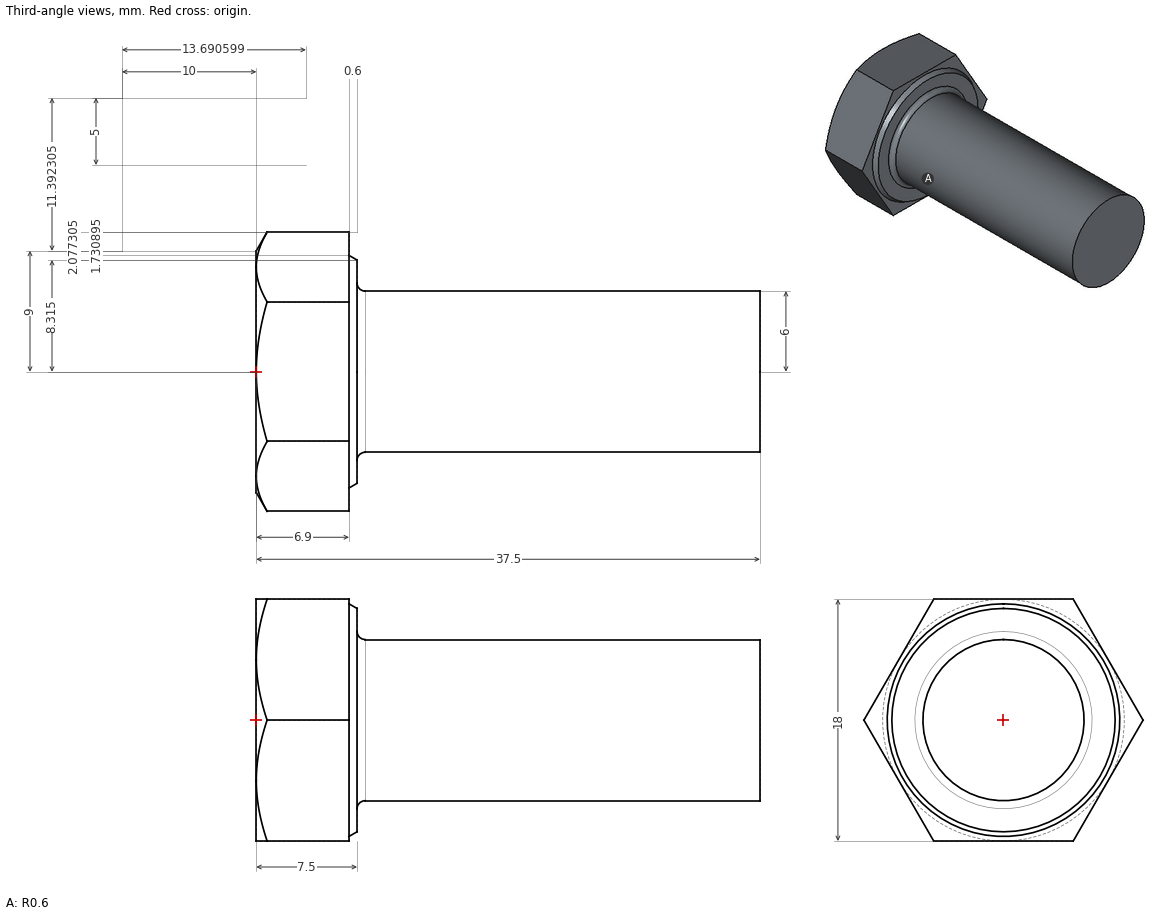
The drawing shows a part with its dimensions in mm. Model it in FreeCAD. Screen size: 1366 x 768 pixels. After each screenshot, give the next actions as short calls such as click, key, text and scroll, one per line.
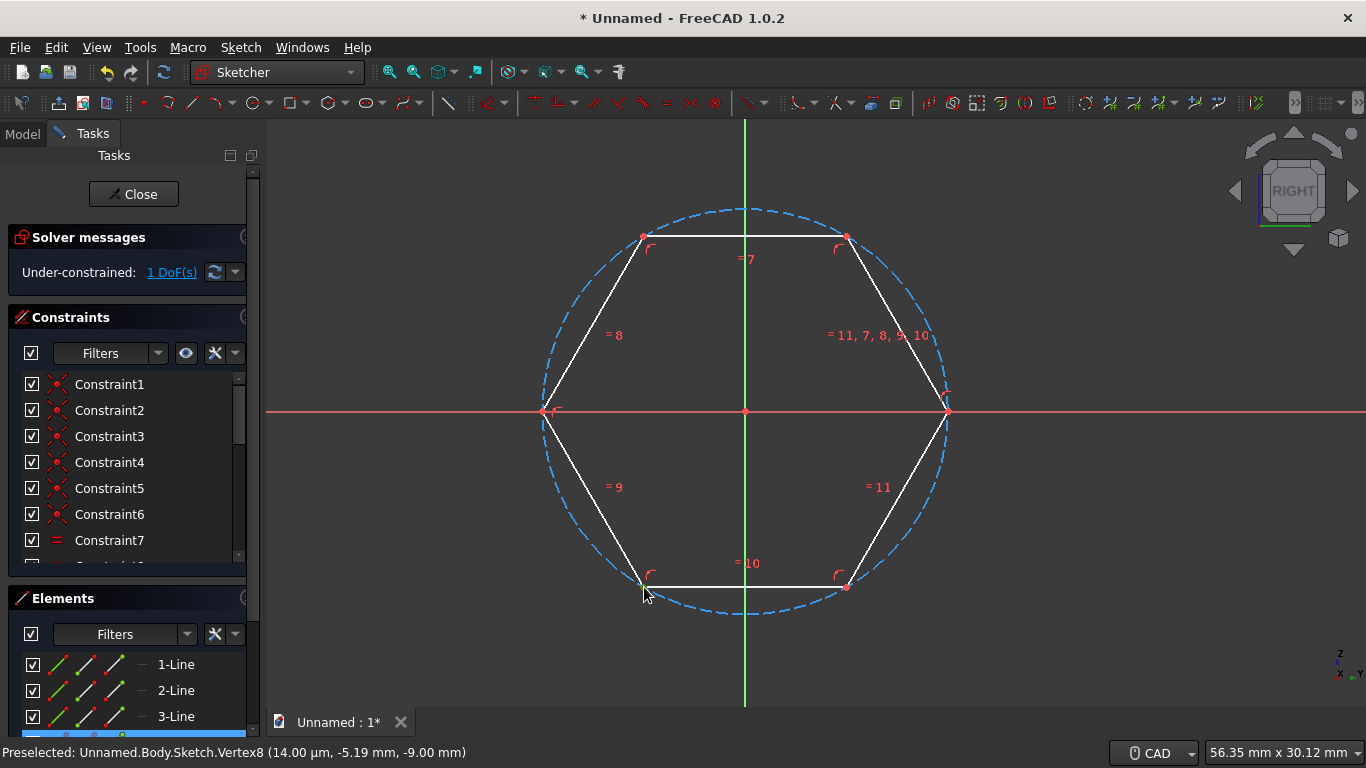
click(847, 236)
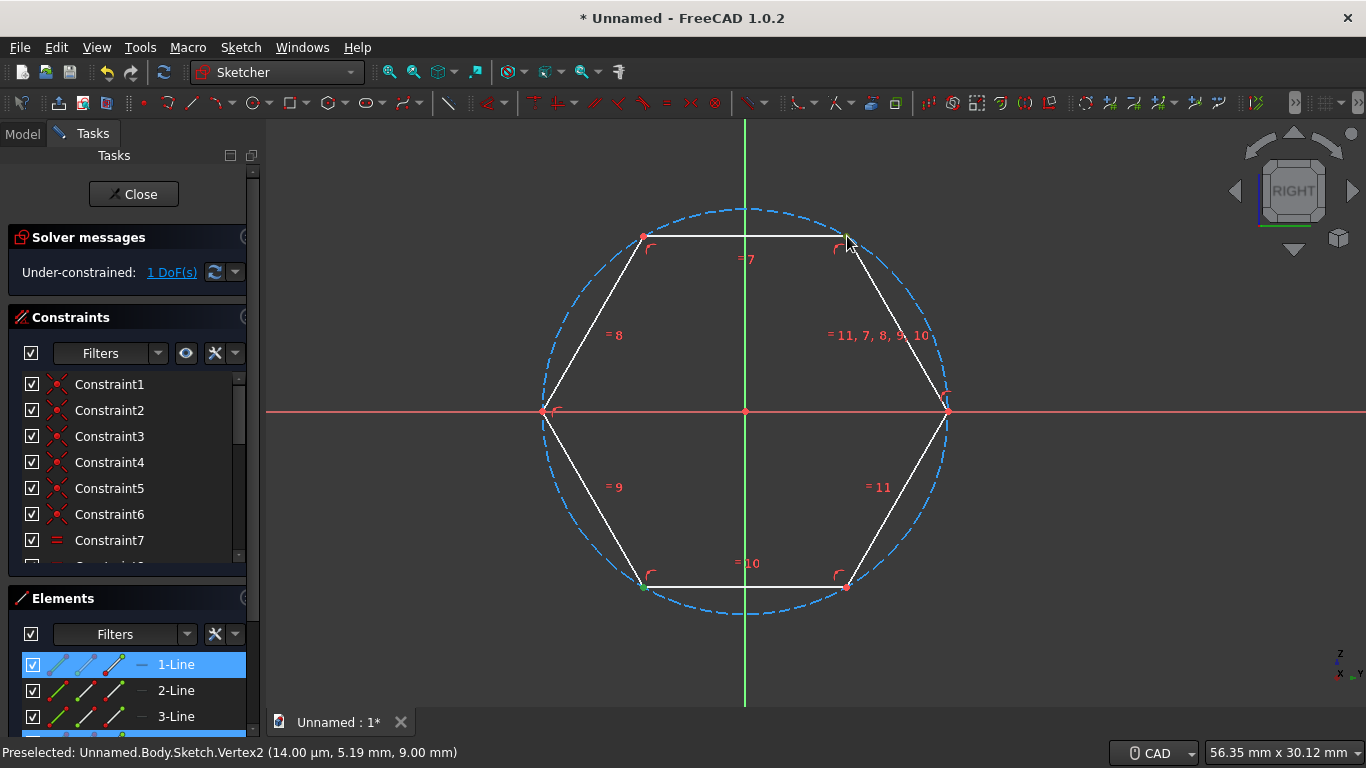
key(i)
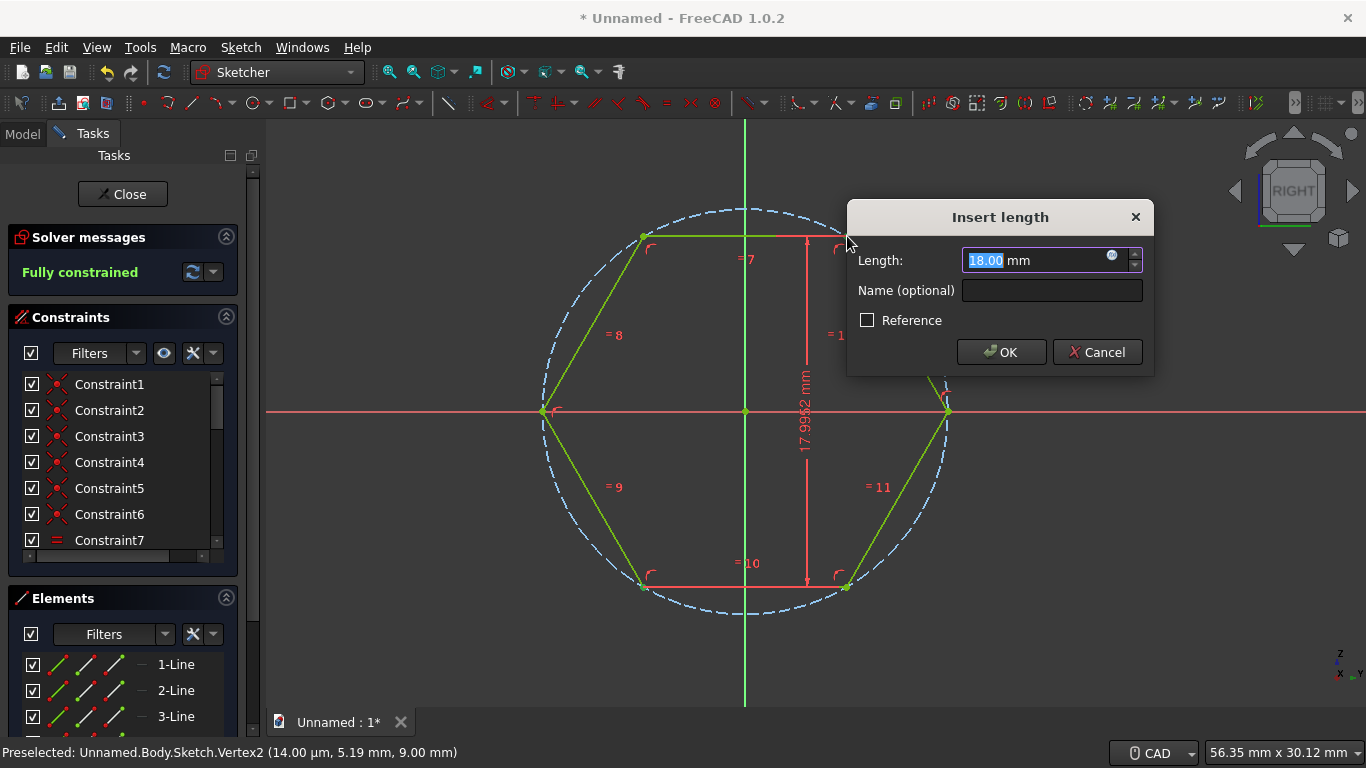
text(18)
key(Return)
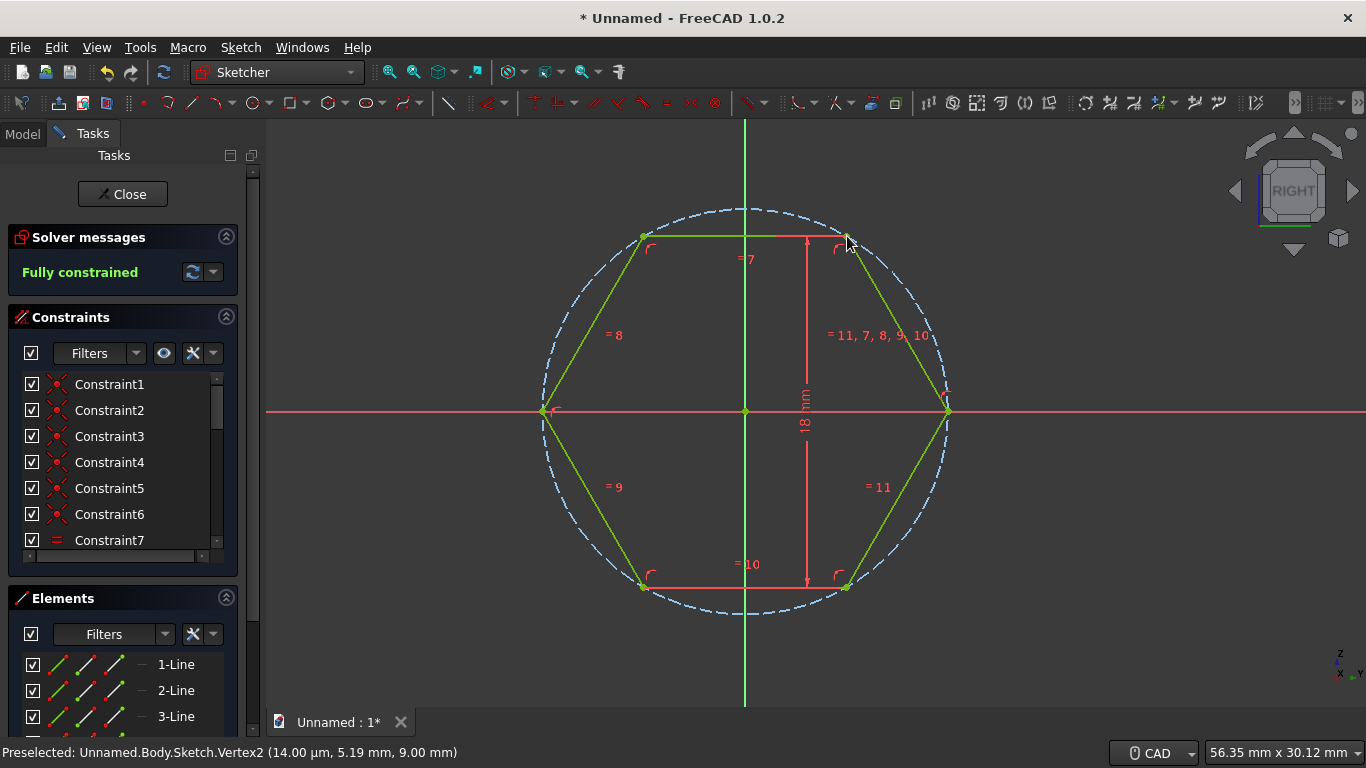
click(123, 194)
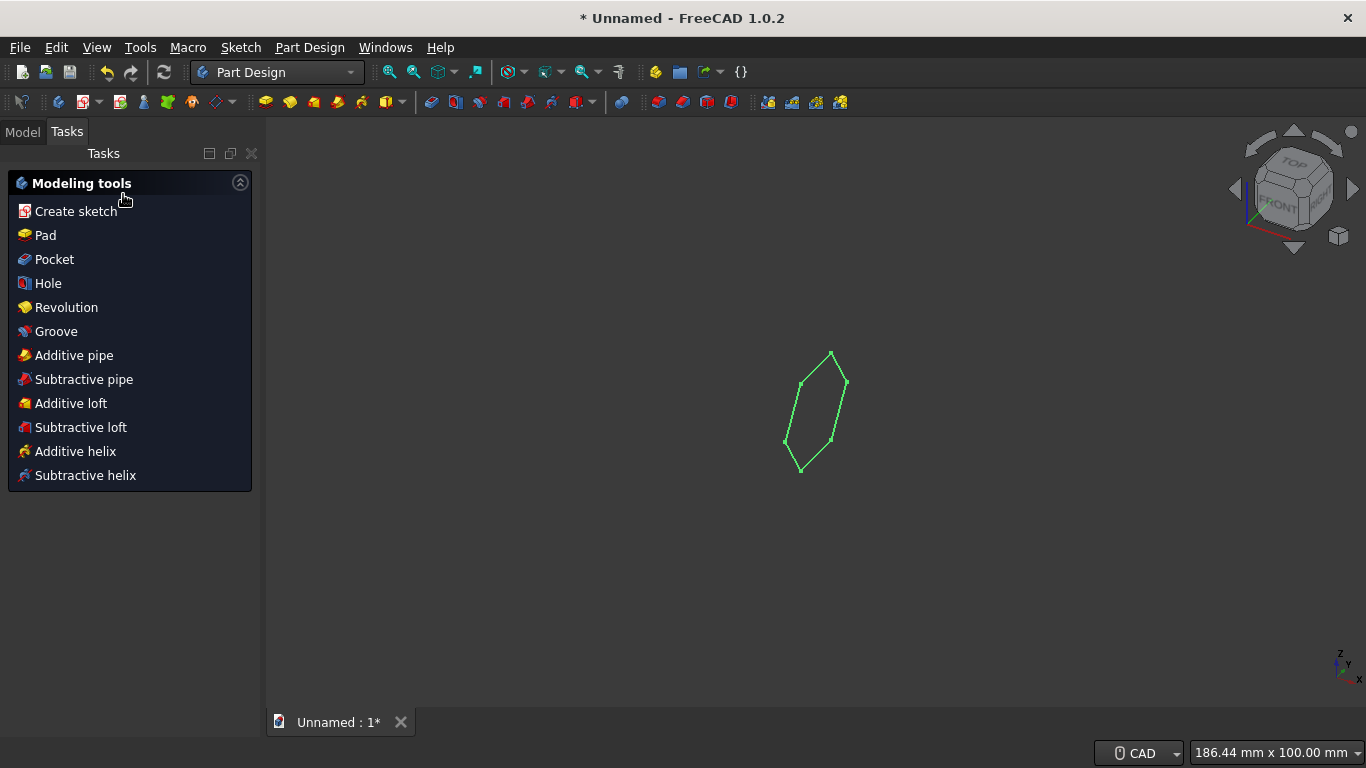
click(266, 102)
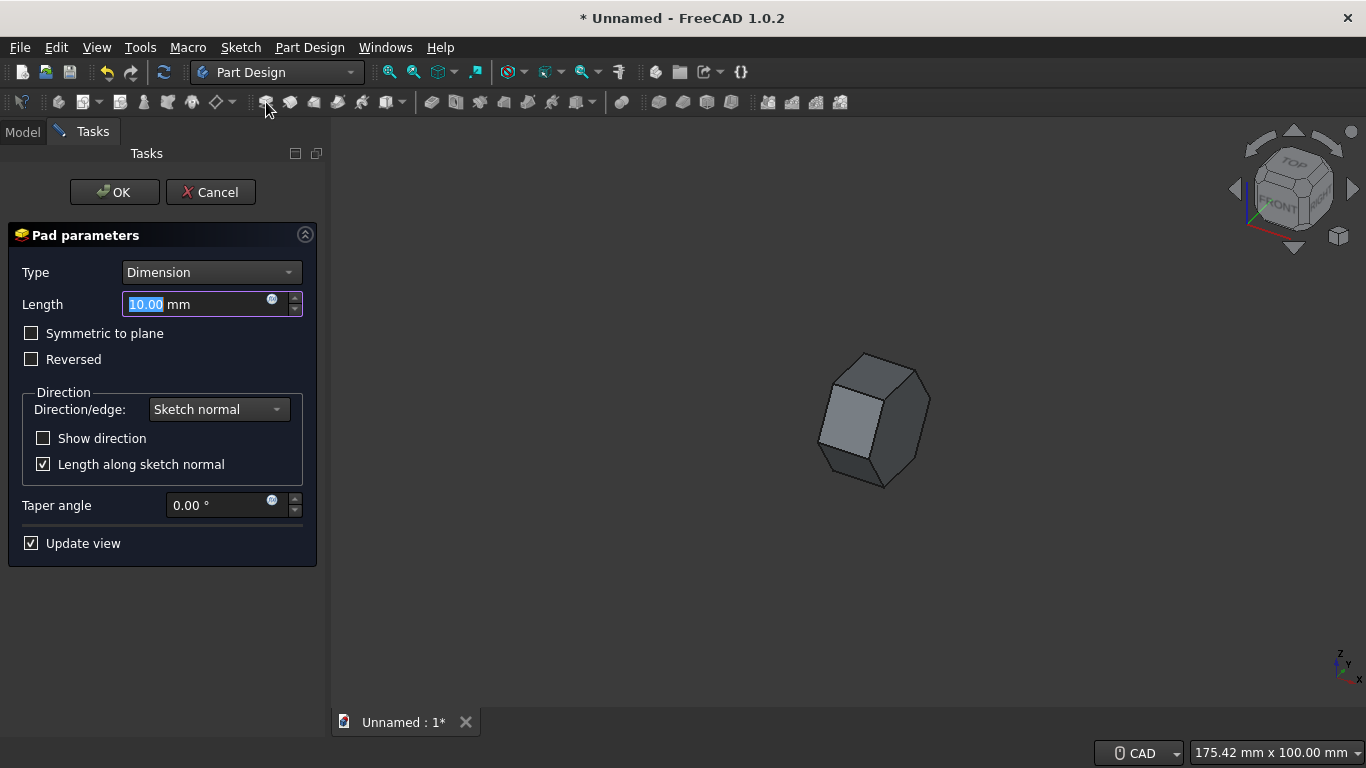
text(7.5)
key(Tab)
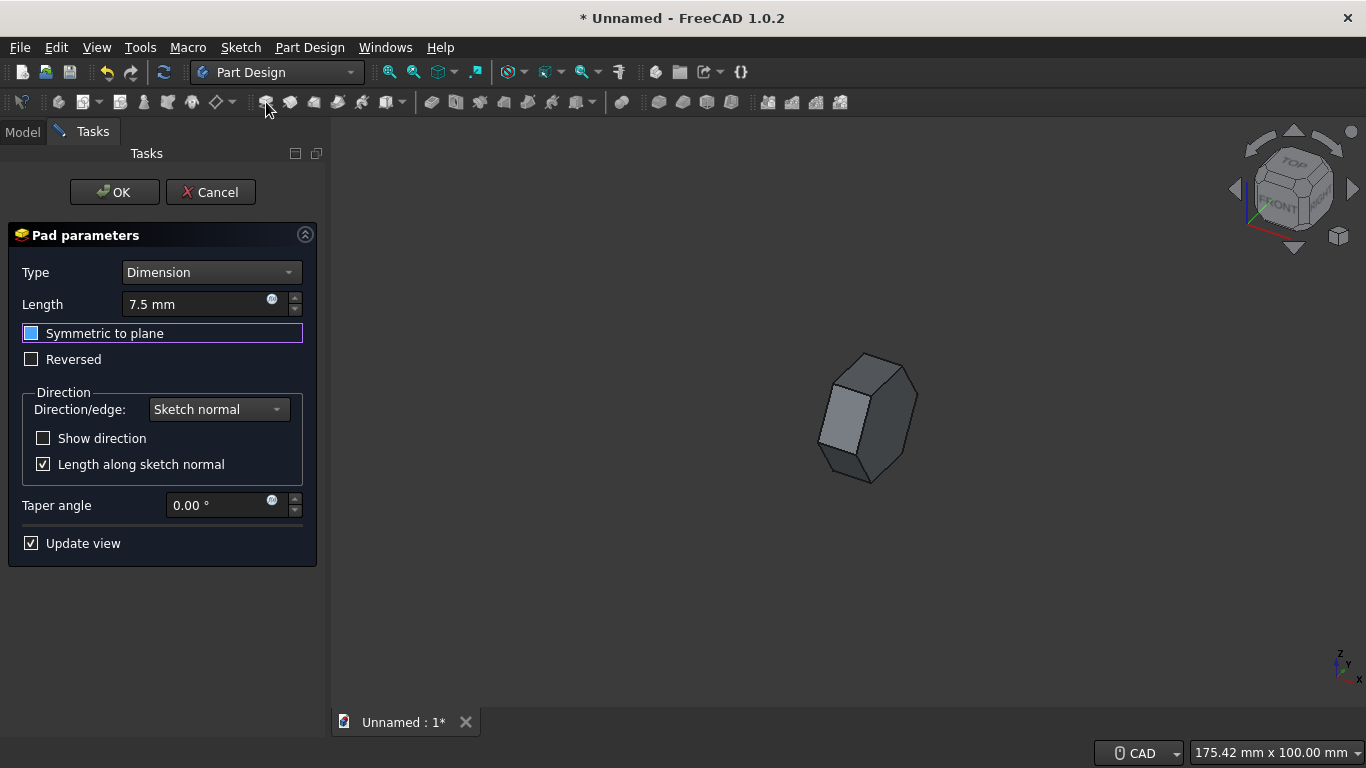
click(115, 192)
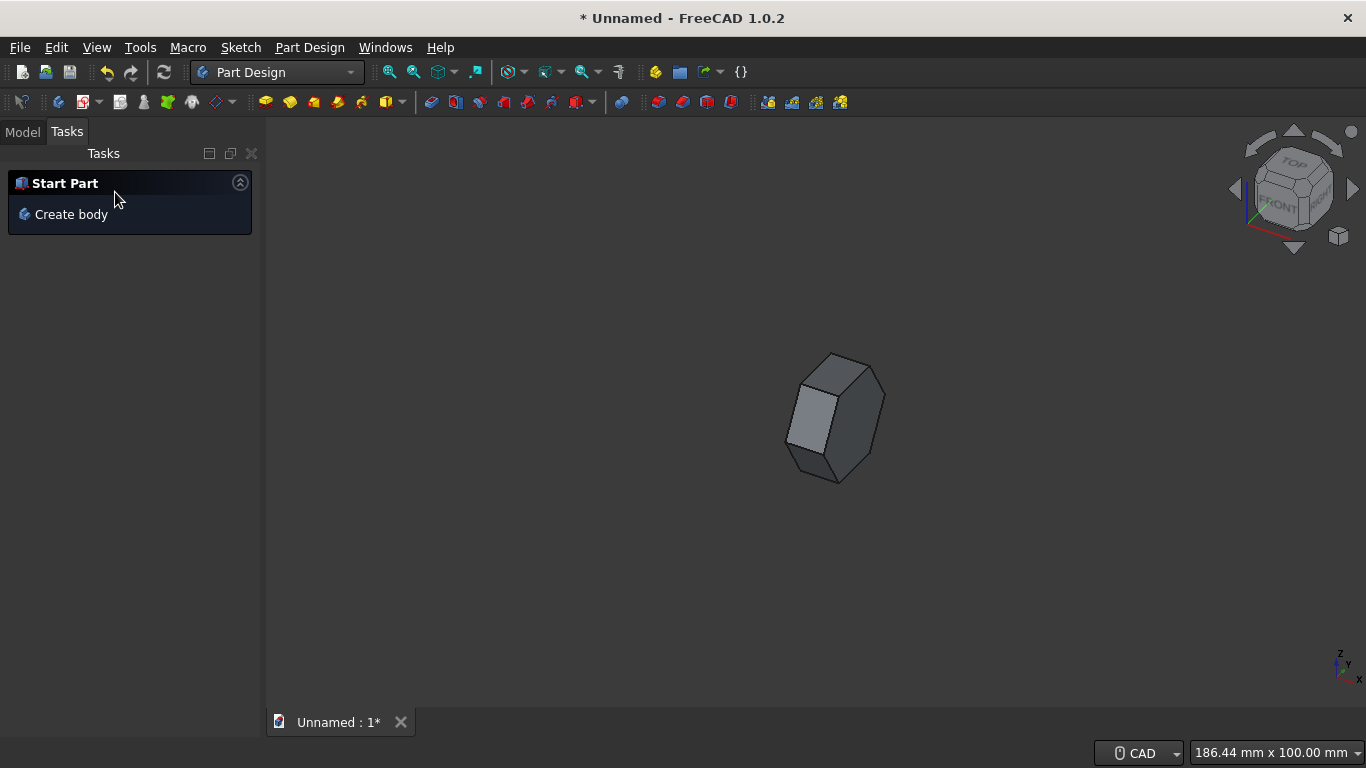
key(v)
key(f)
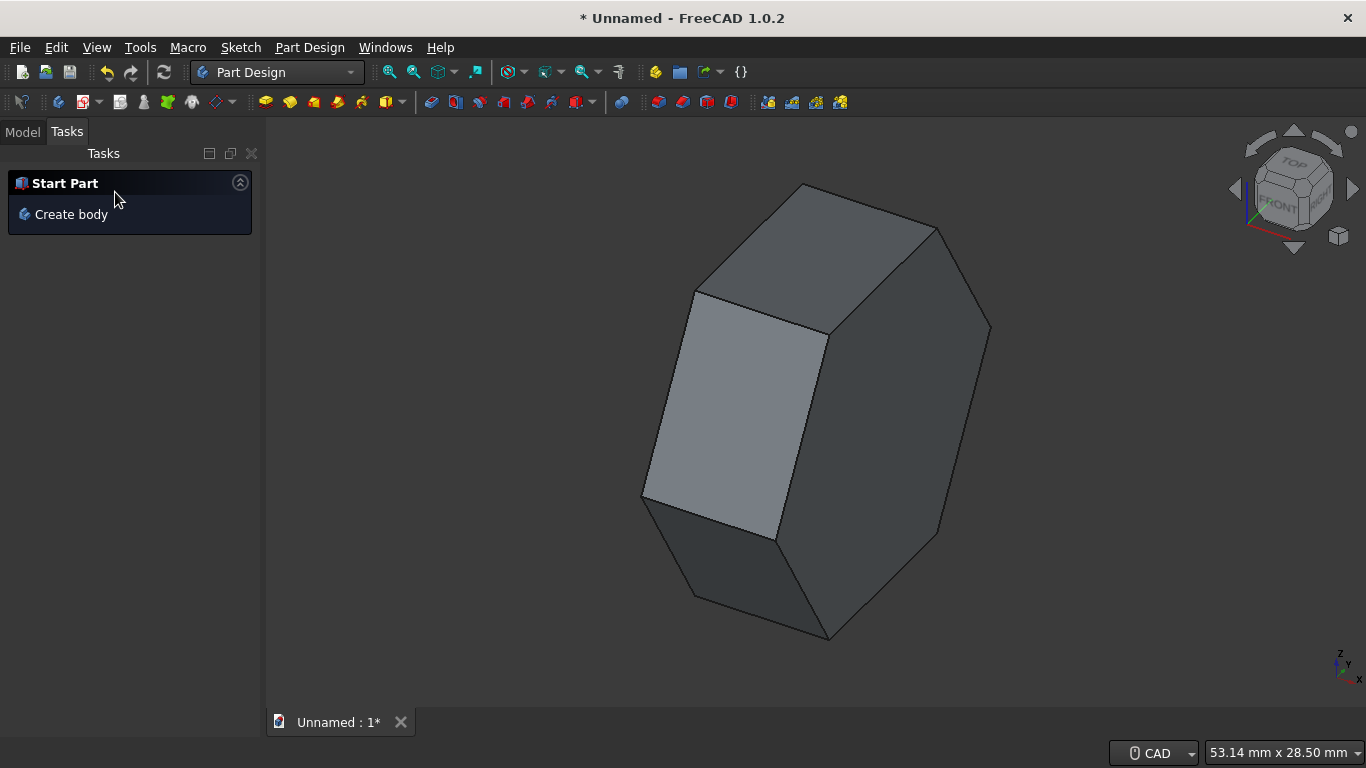
click(84, 102)